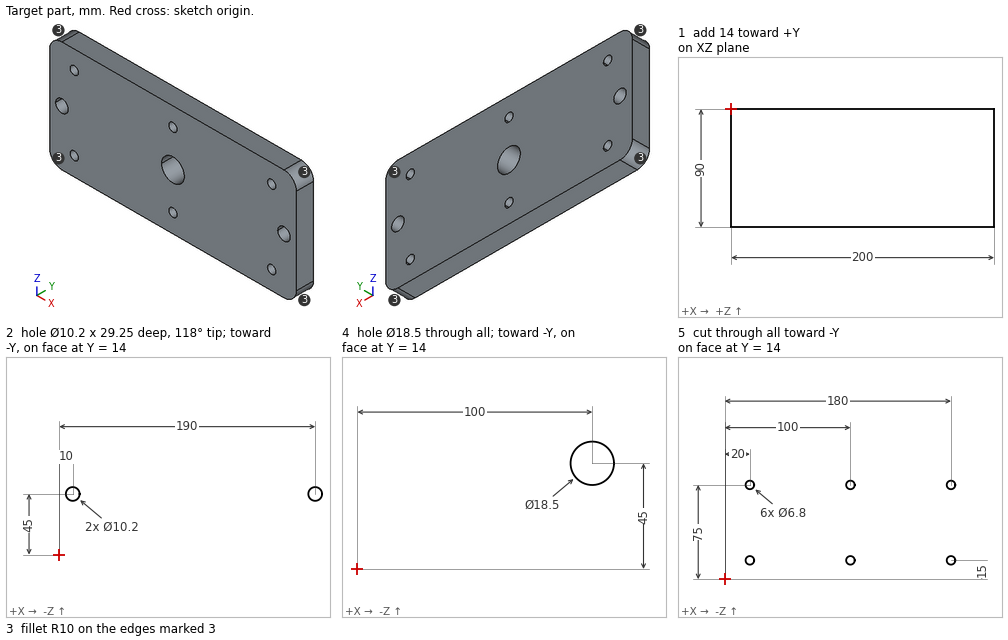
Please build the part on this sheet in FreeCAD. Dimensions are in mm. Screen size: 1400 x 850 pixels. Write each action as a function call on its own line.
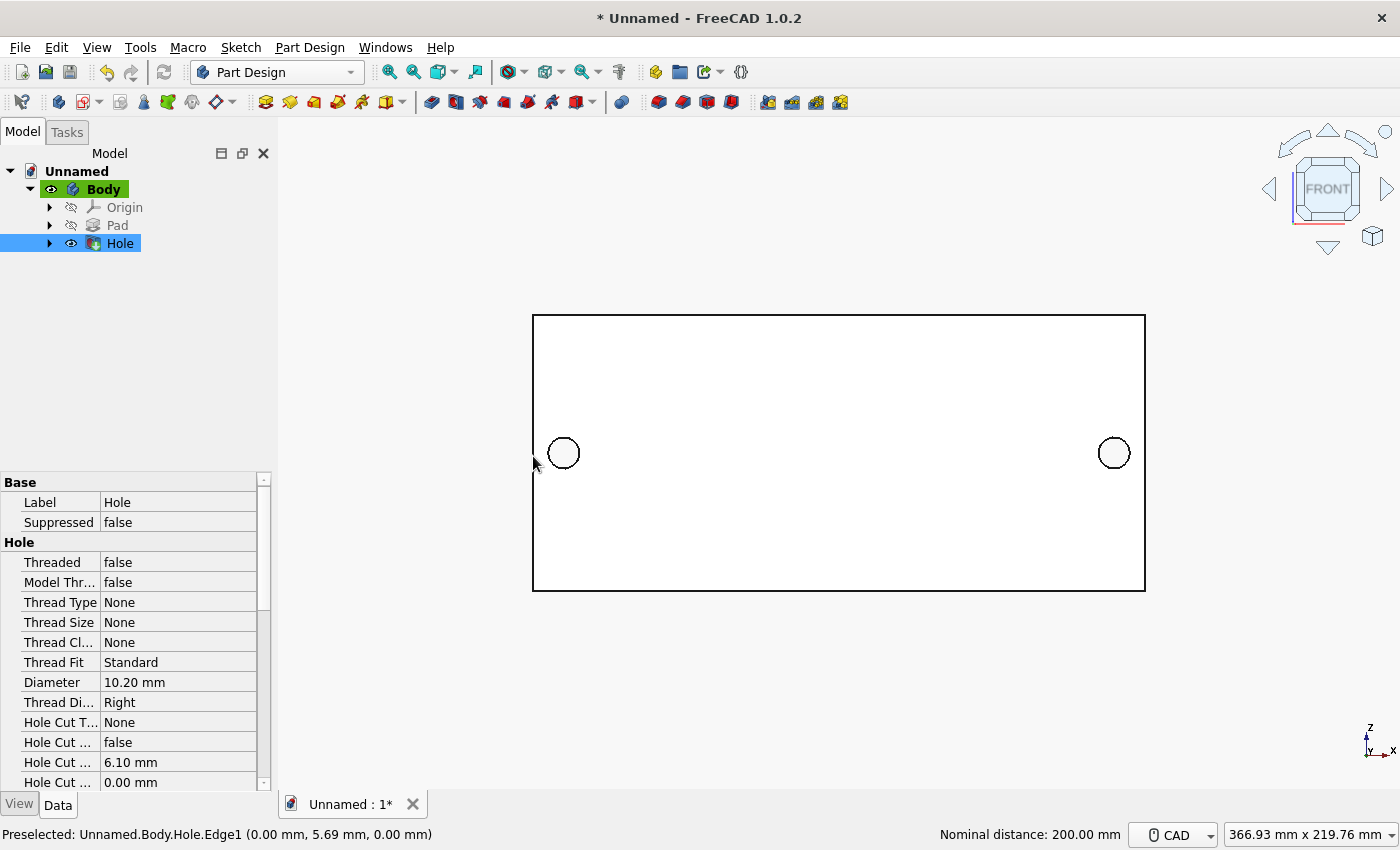
key(3)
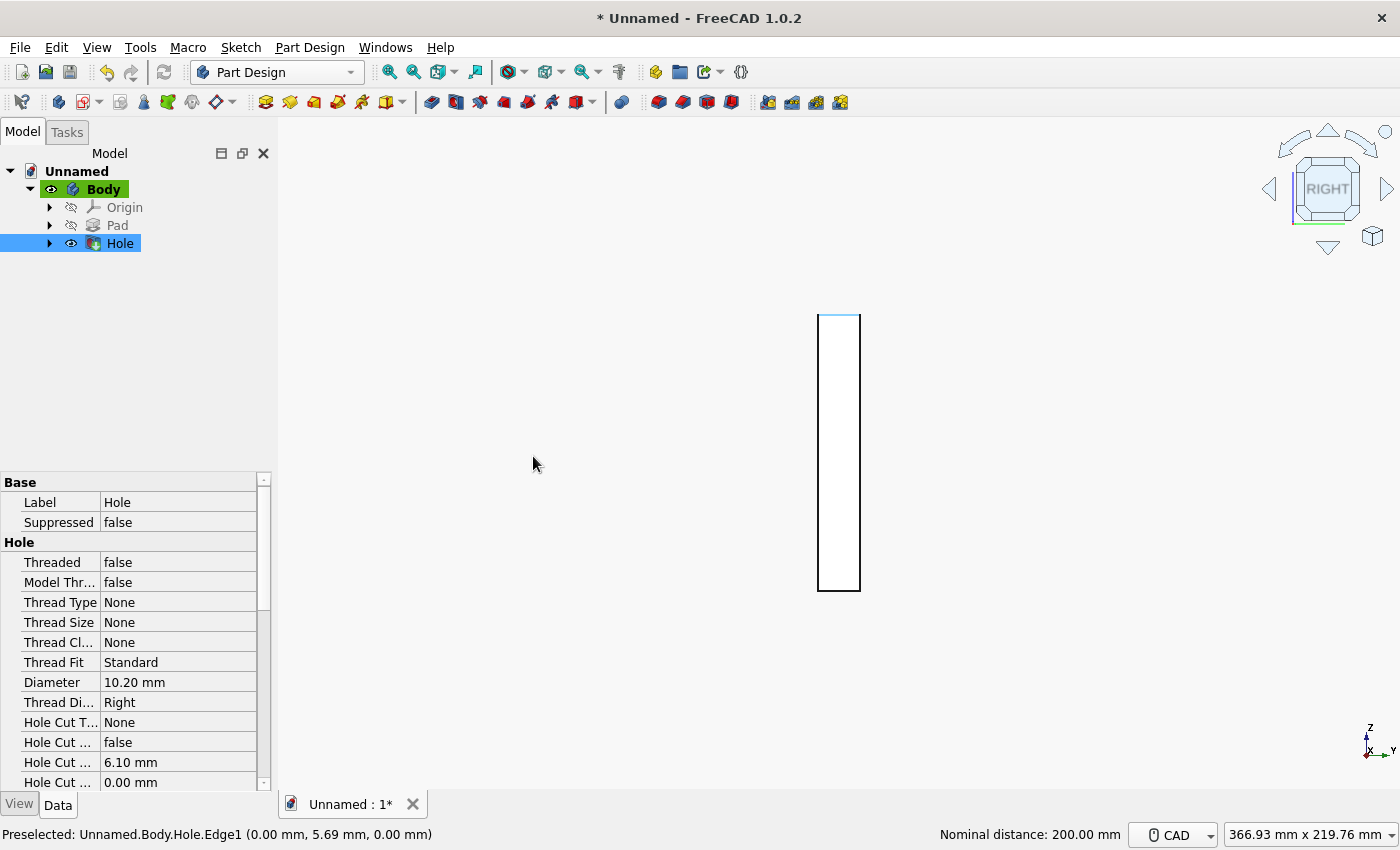
click(390, 72)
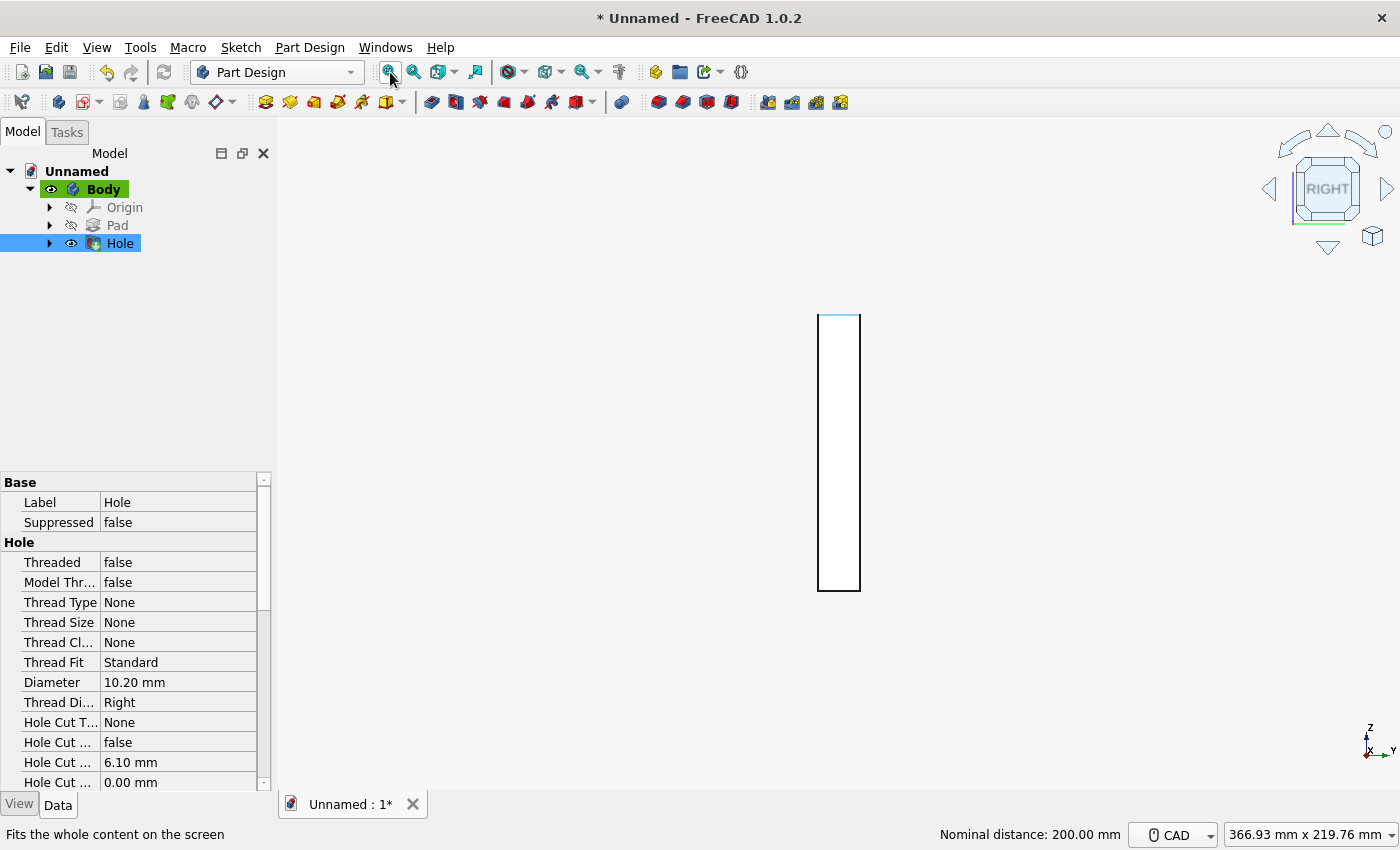
click(839, 590, ctrl)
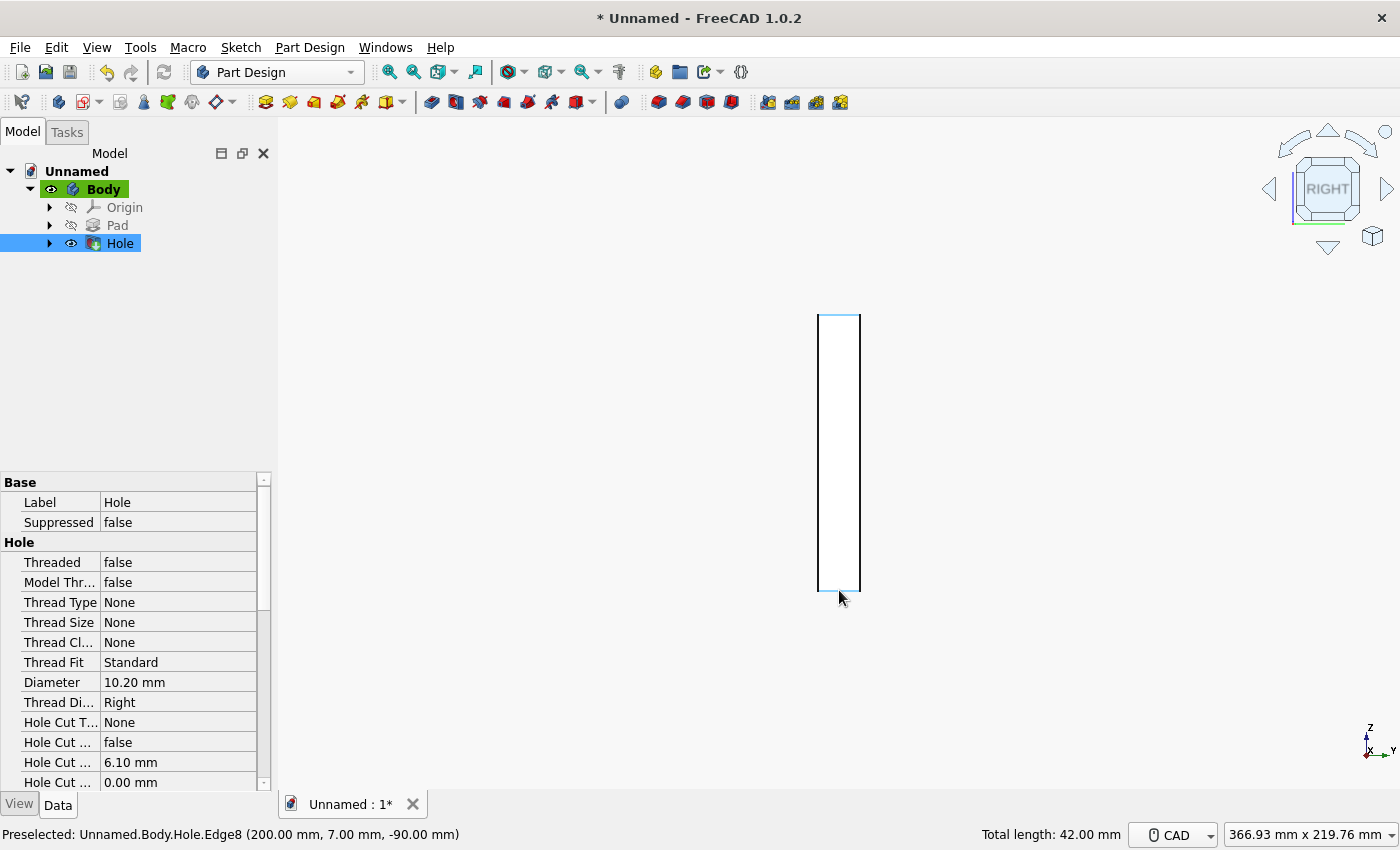
key(5)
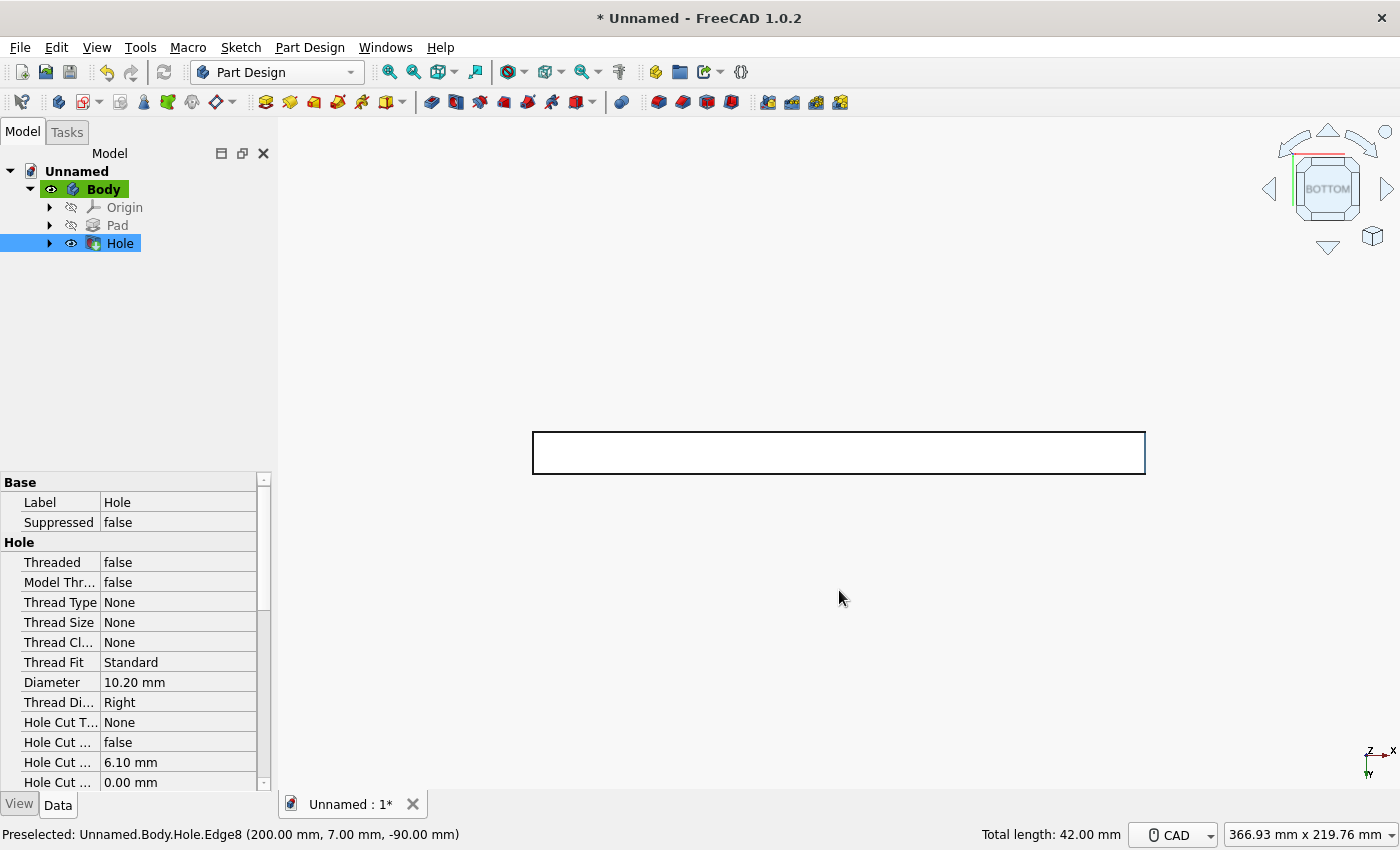
click(533, 452, ctrl)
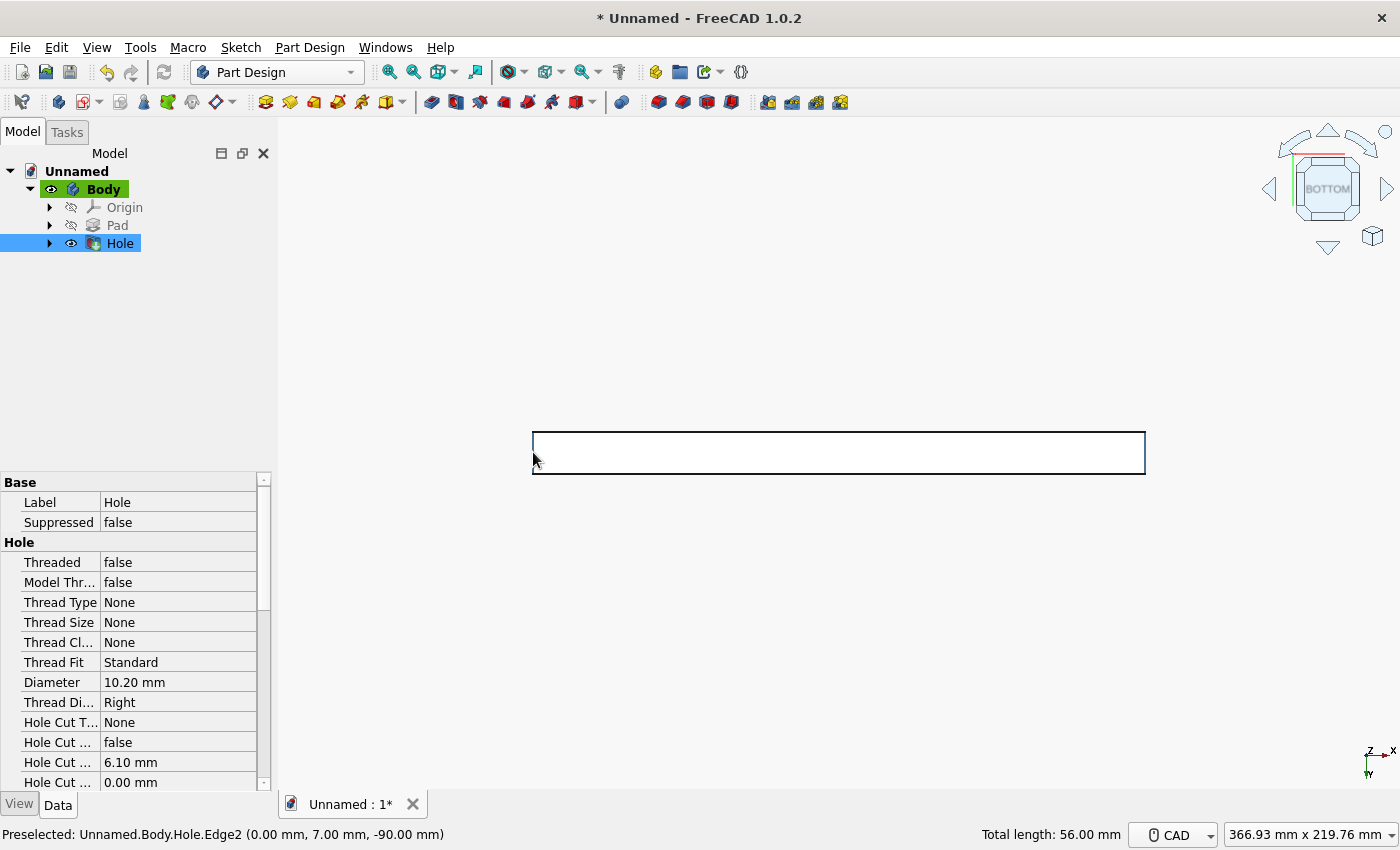
click(660, 102)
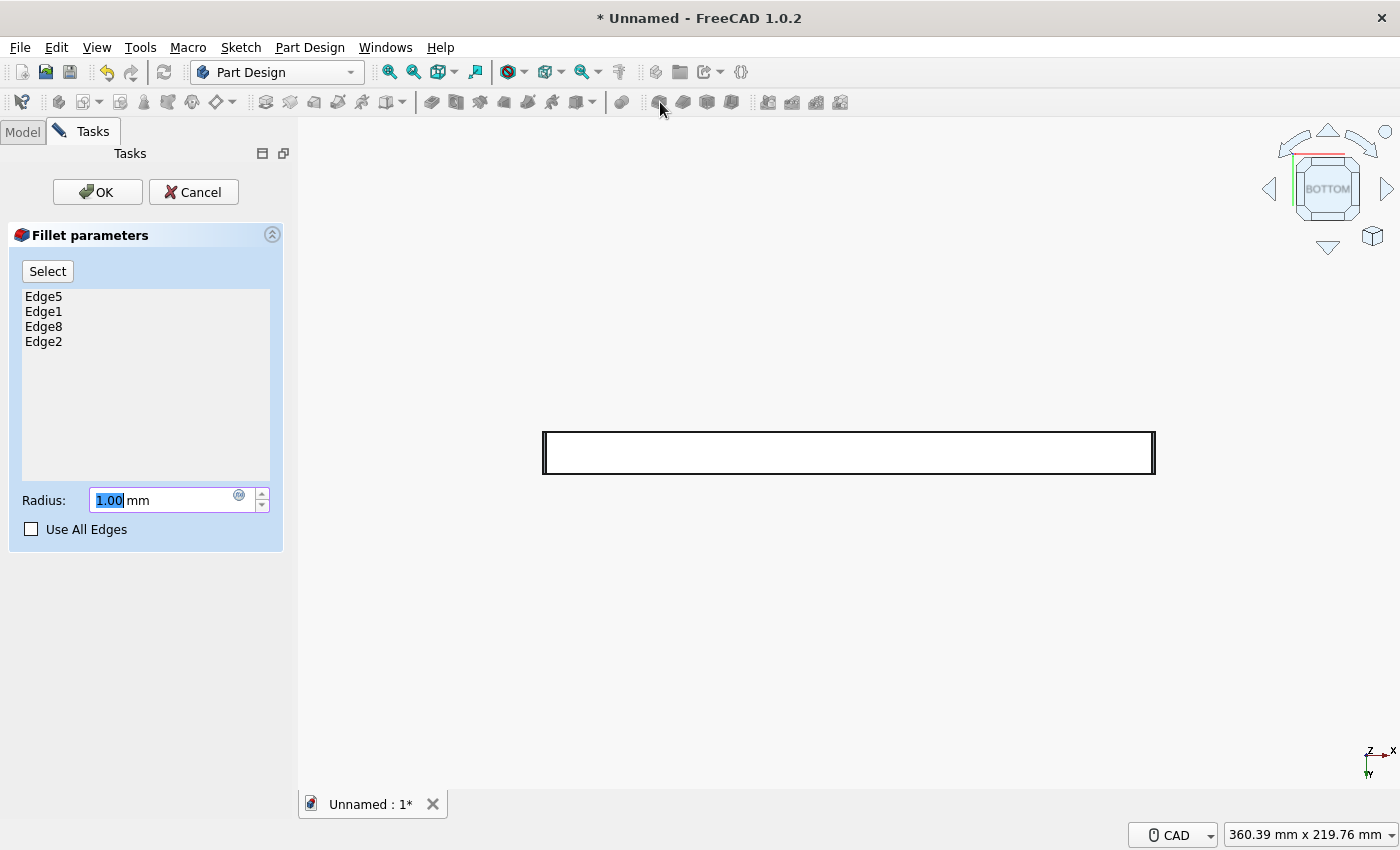
text(10)
key(Tab)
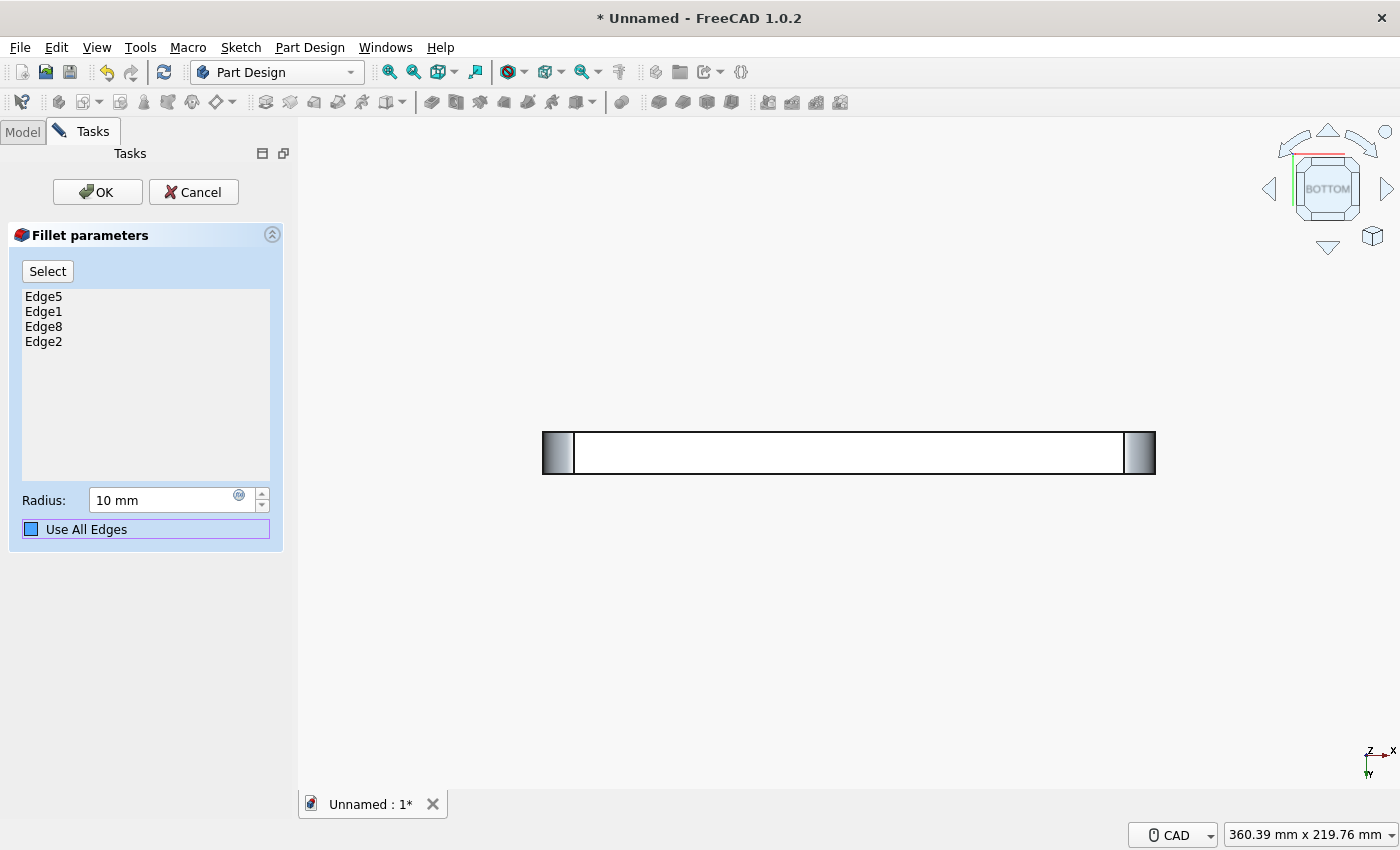
click(98, 192)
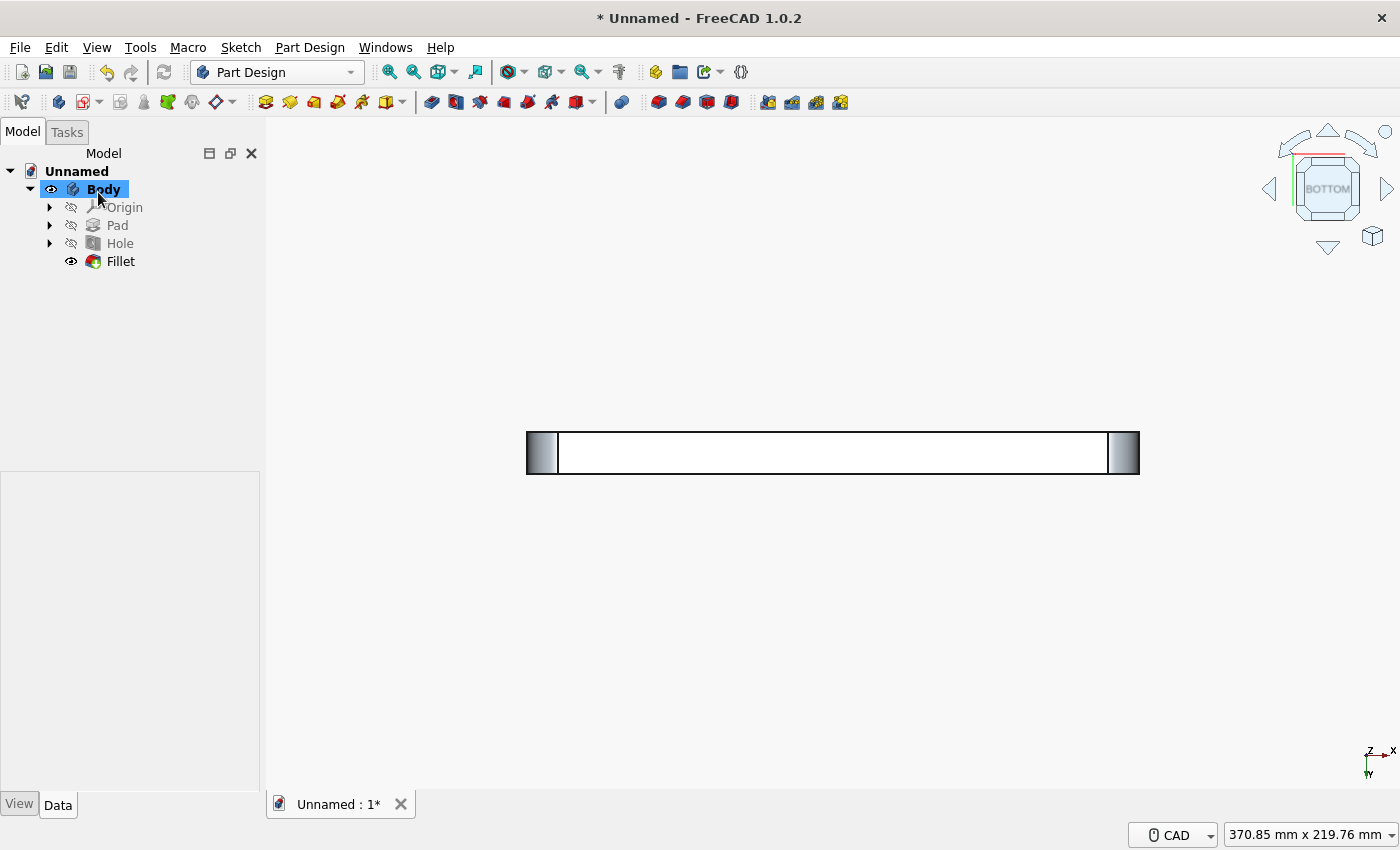
key(4)